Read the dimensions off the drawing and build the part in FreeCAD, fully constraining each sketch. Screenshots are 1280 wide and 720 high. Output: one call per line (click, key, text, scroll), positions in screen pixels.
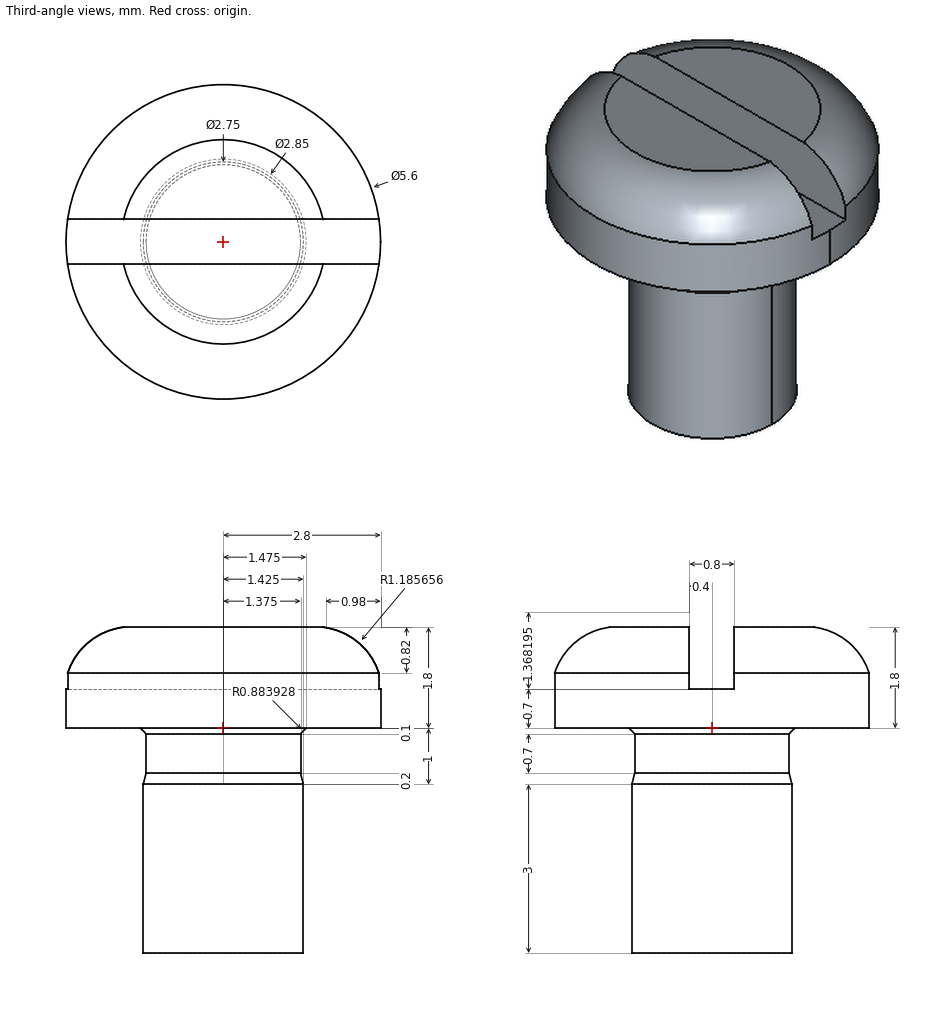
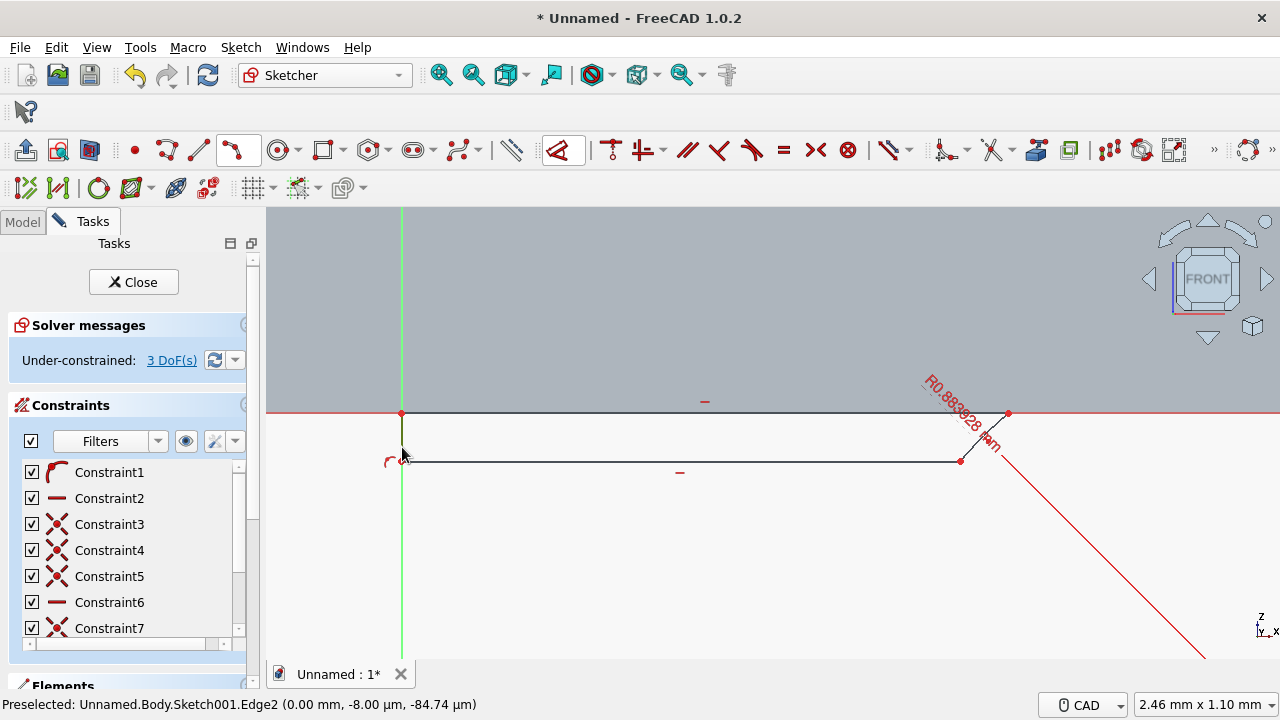
click(580, 150)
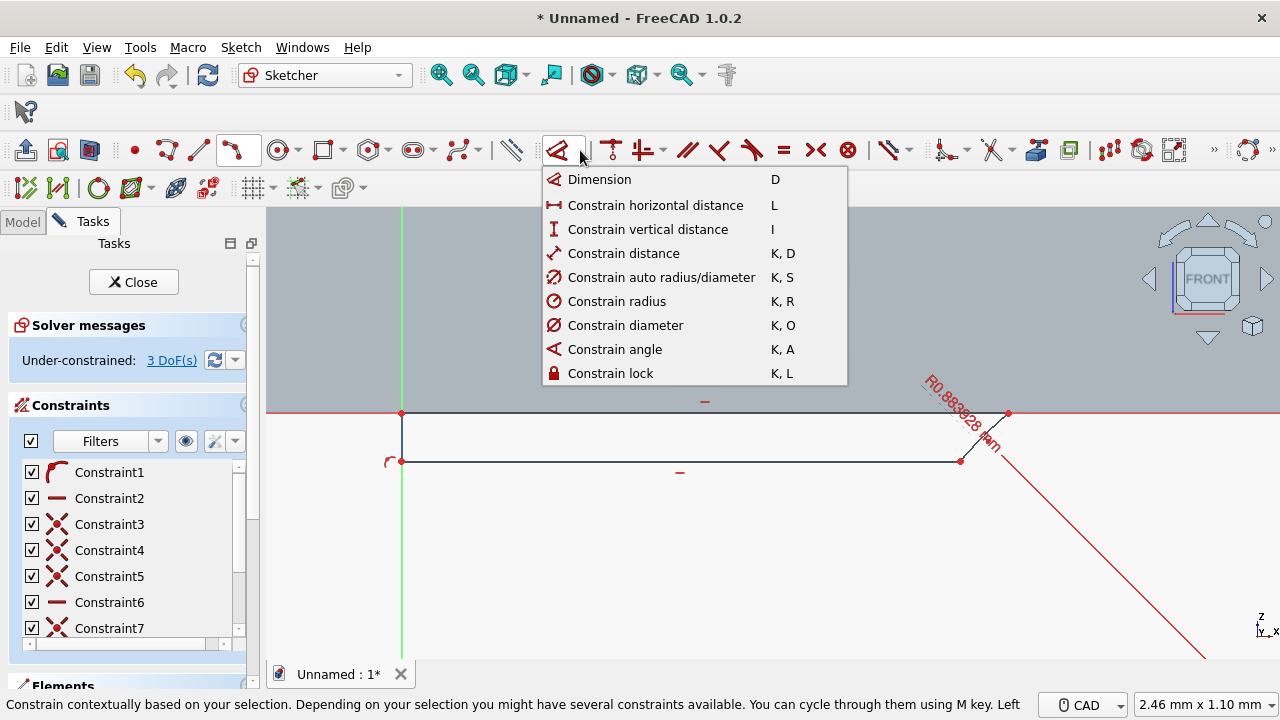
click(695, 229)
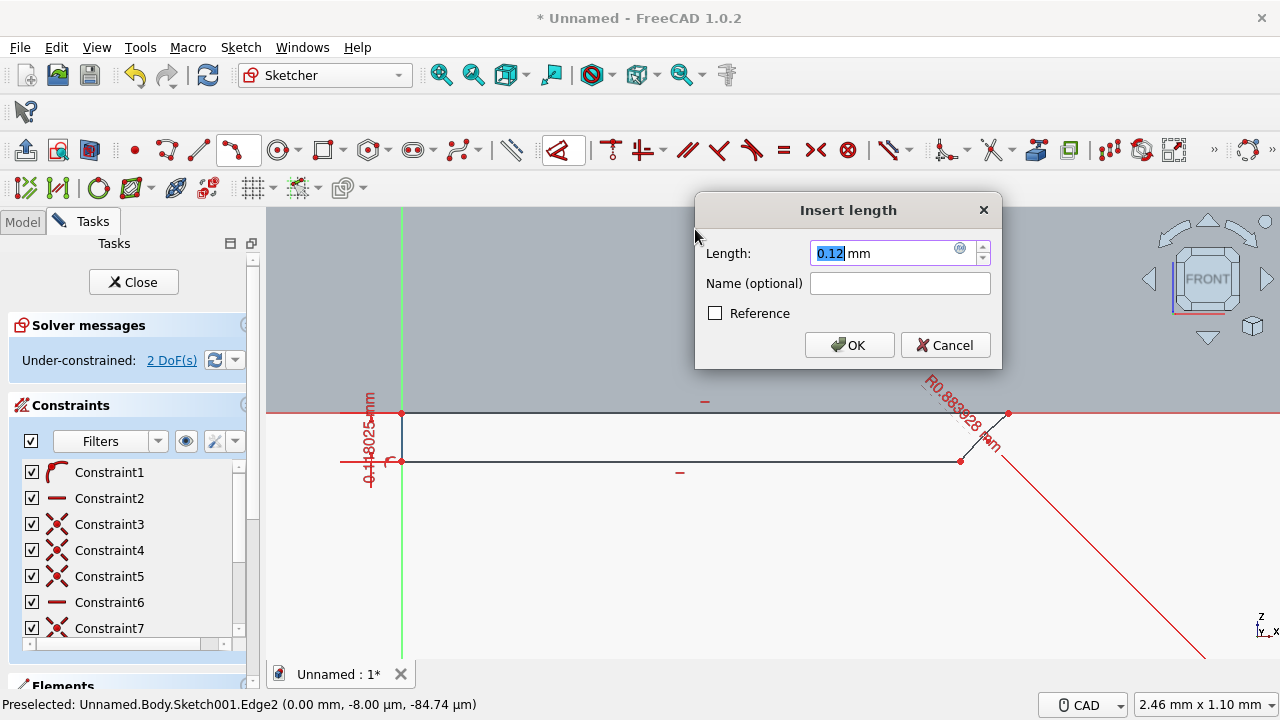
text(0.1)
key(Return)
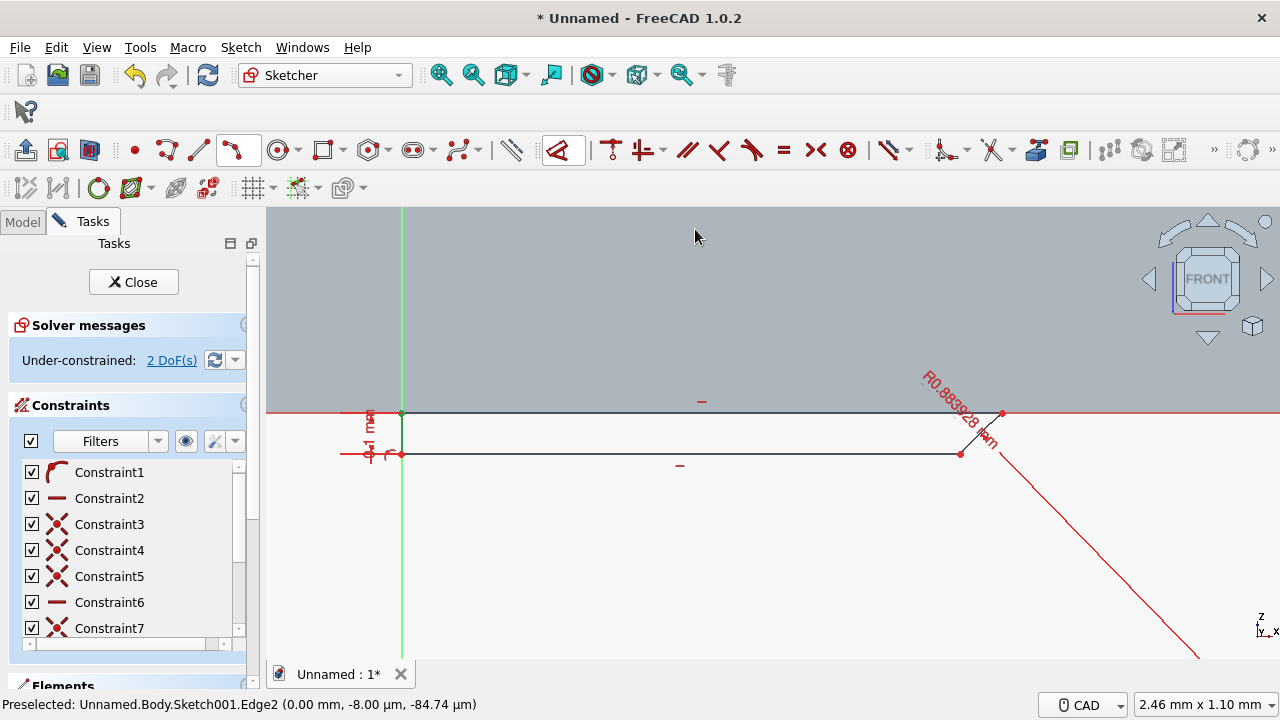
click(793, 454)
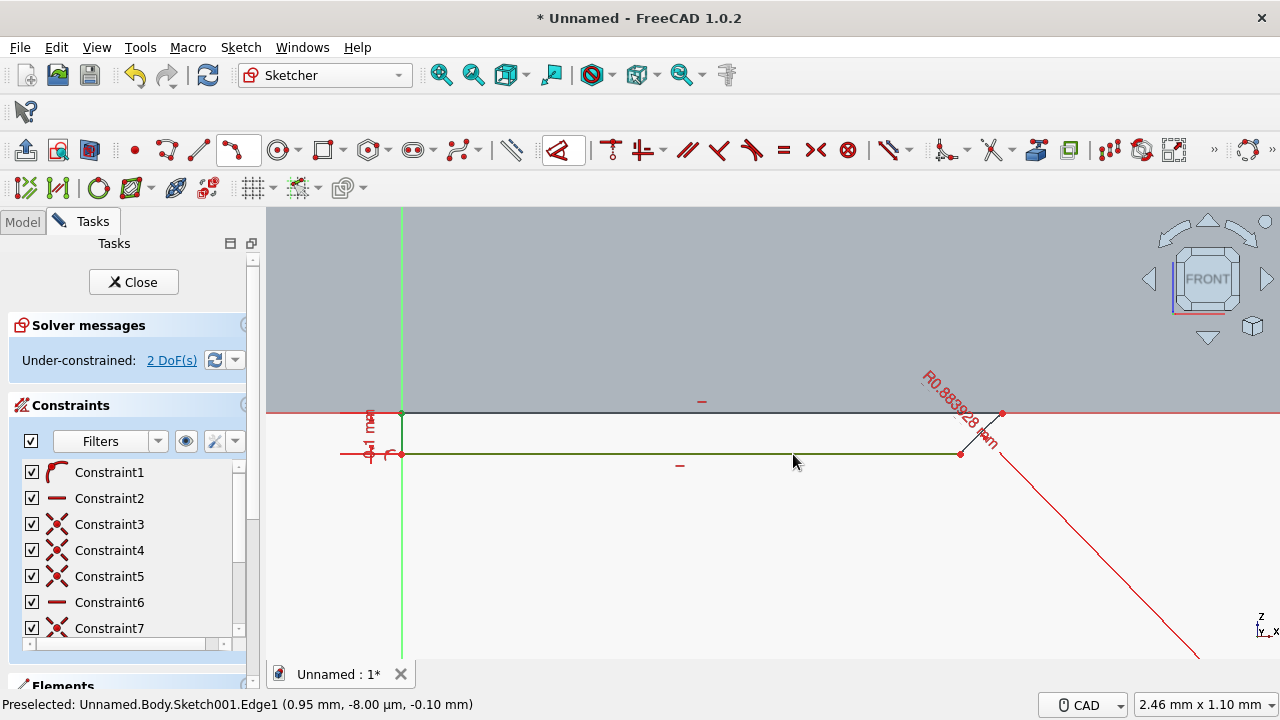
click(580, 150)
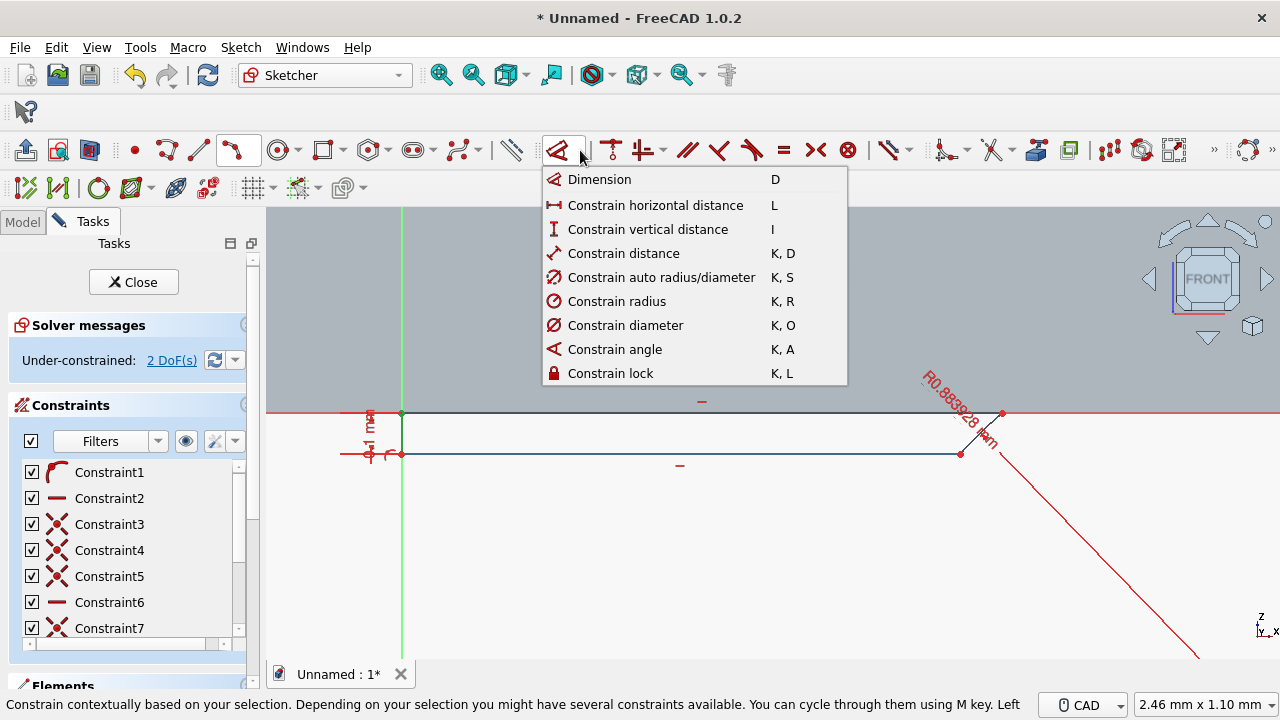
click(695, 205)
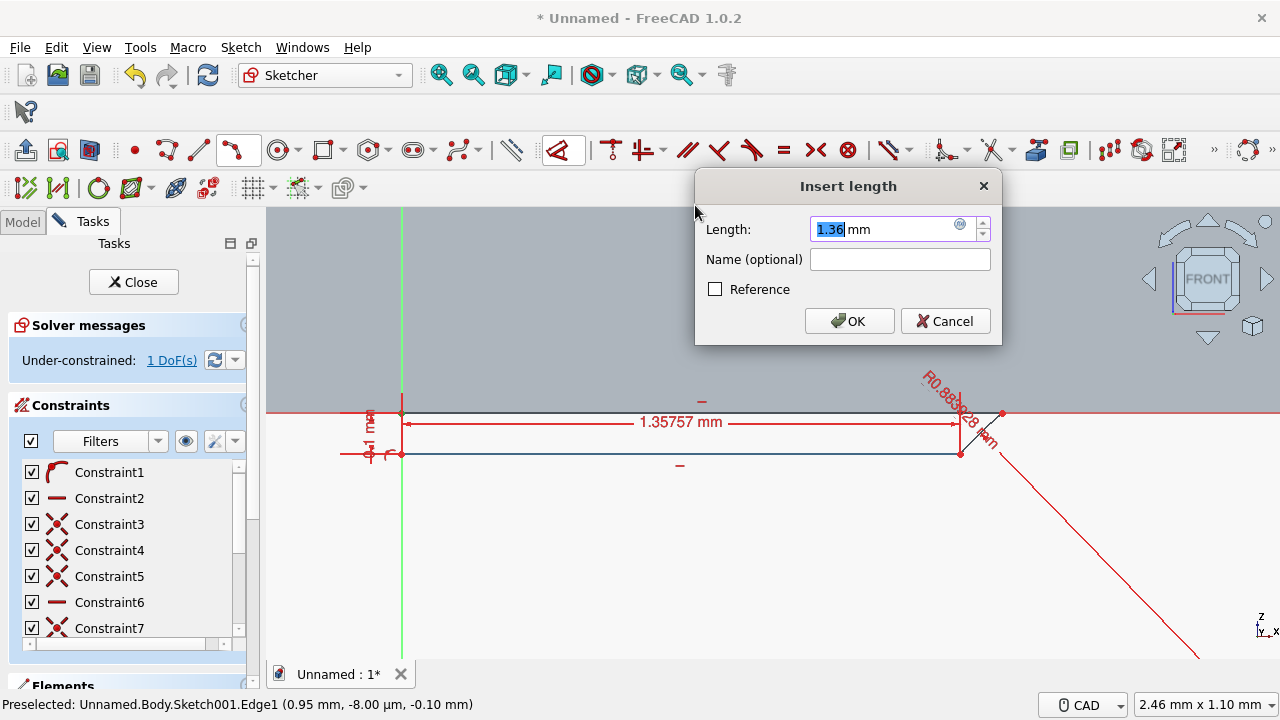
text(1.375)
key(Return)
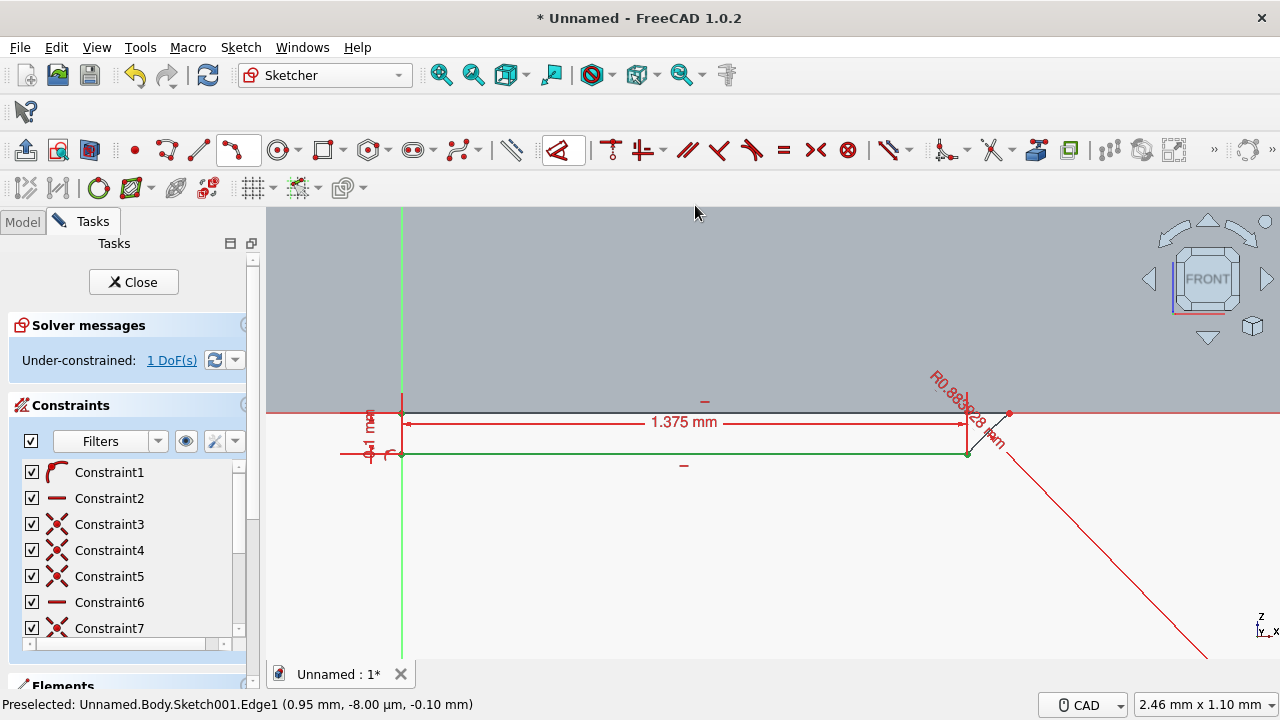
click(1010, 413)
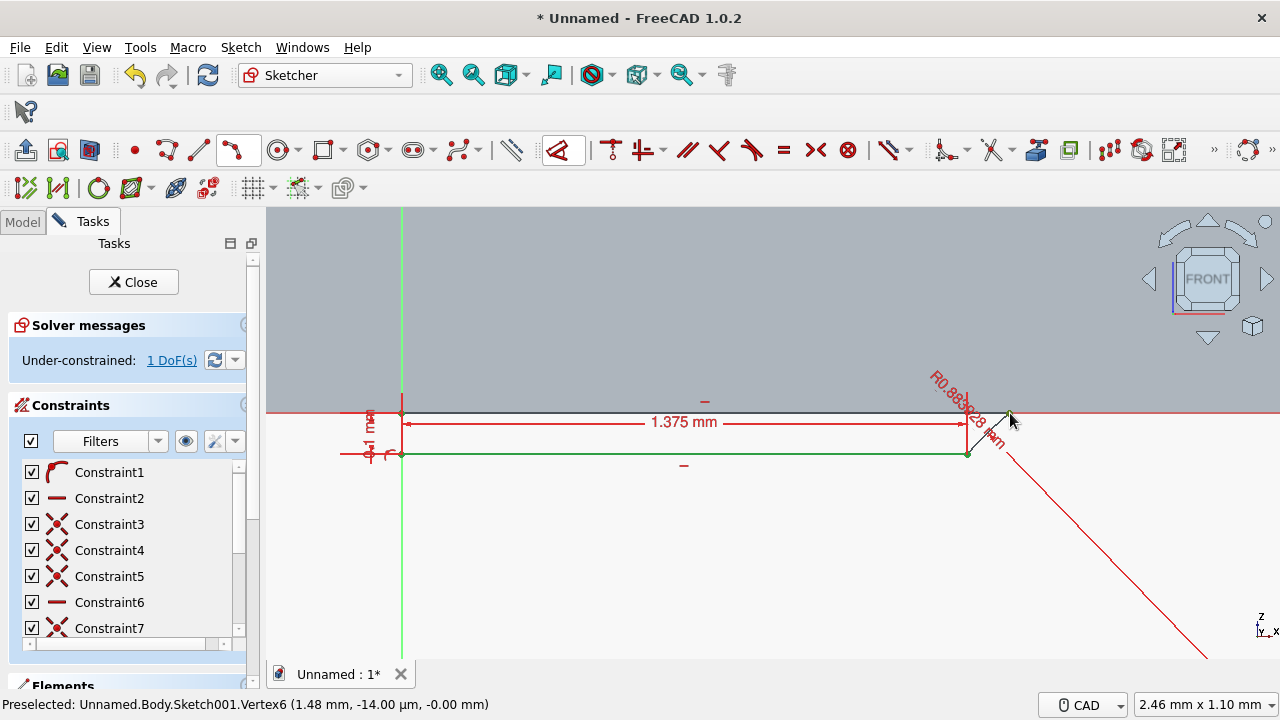
click(580, 150)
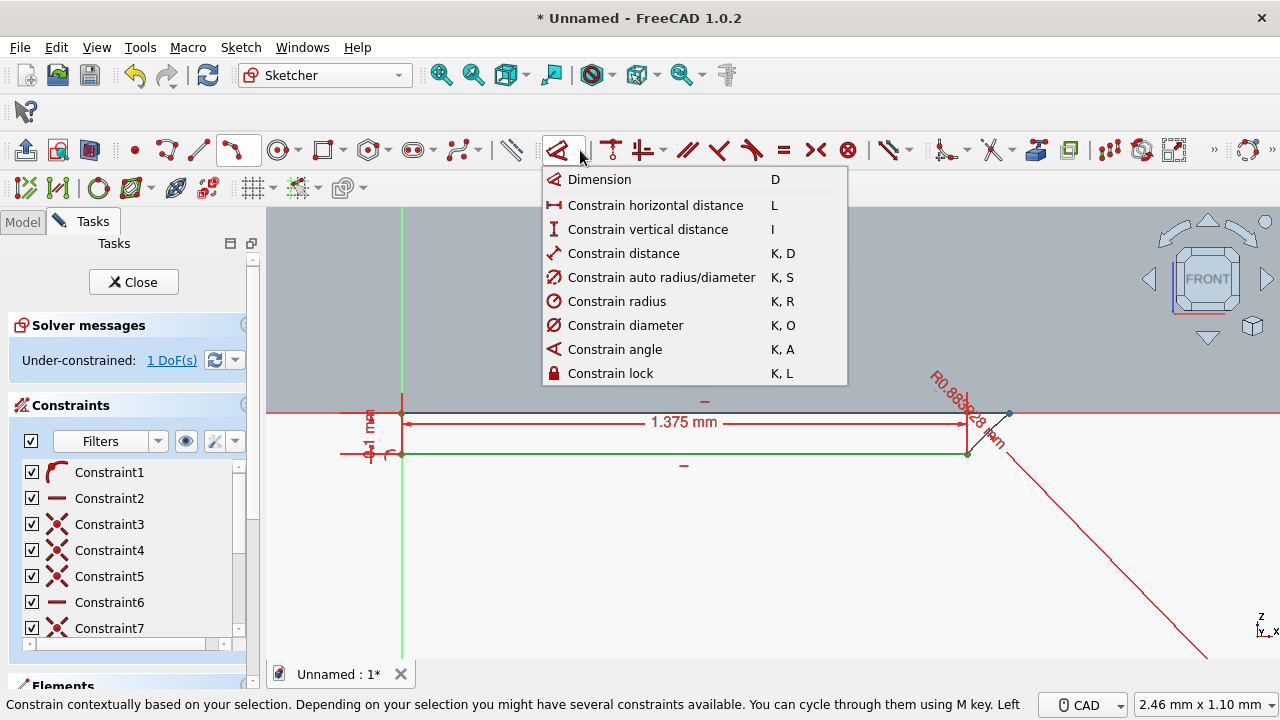
click(695, 205)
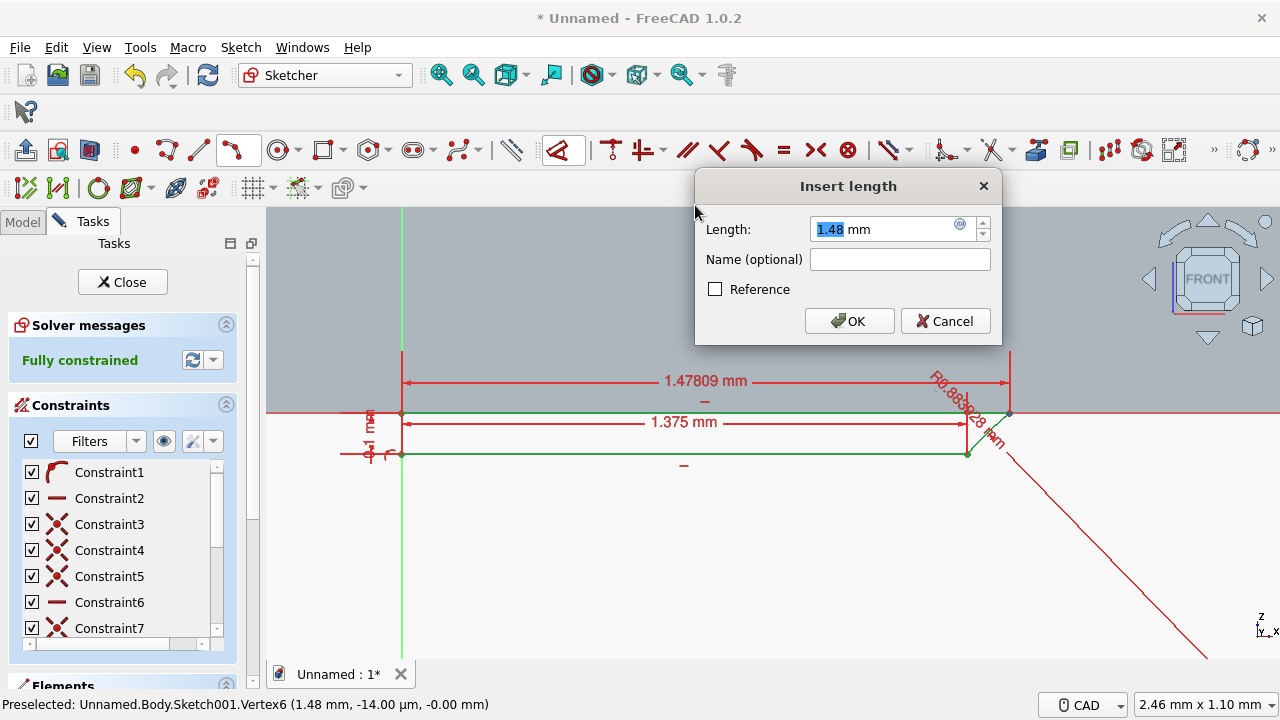
text(1.475)
key(Return)